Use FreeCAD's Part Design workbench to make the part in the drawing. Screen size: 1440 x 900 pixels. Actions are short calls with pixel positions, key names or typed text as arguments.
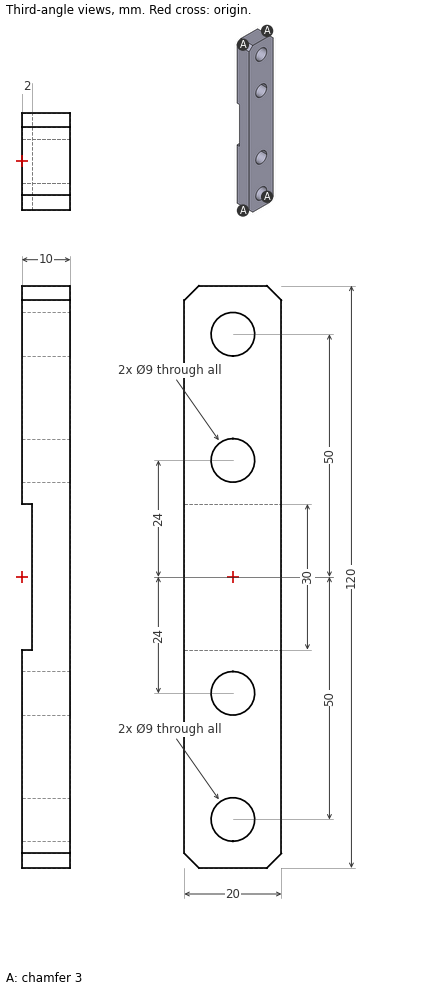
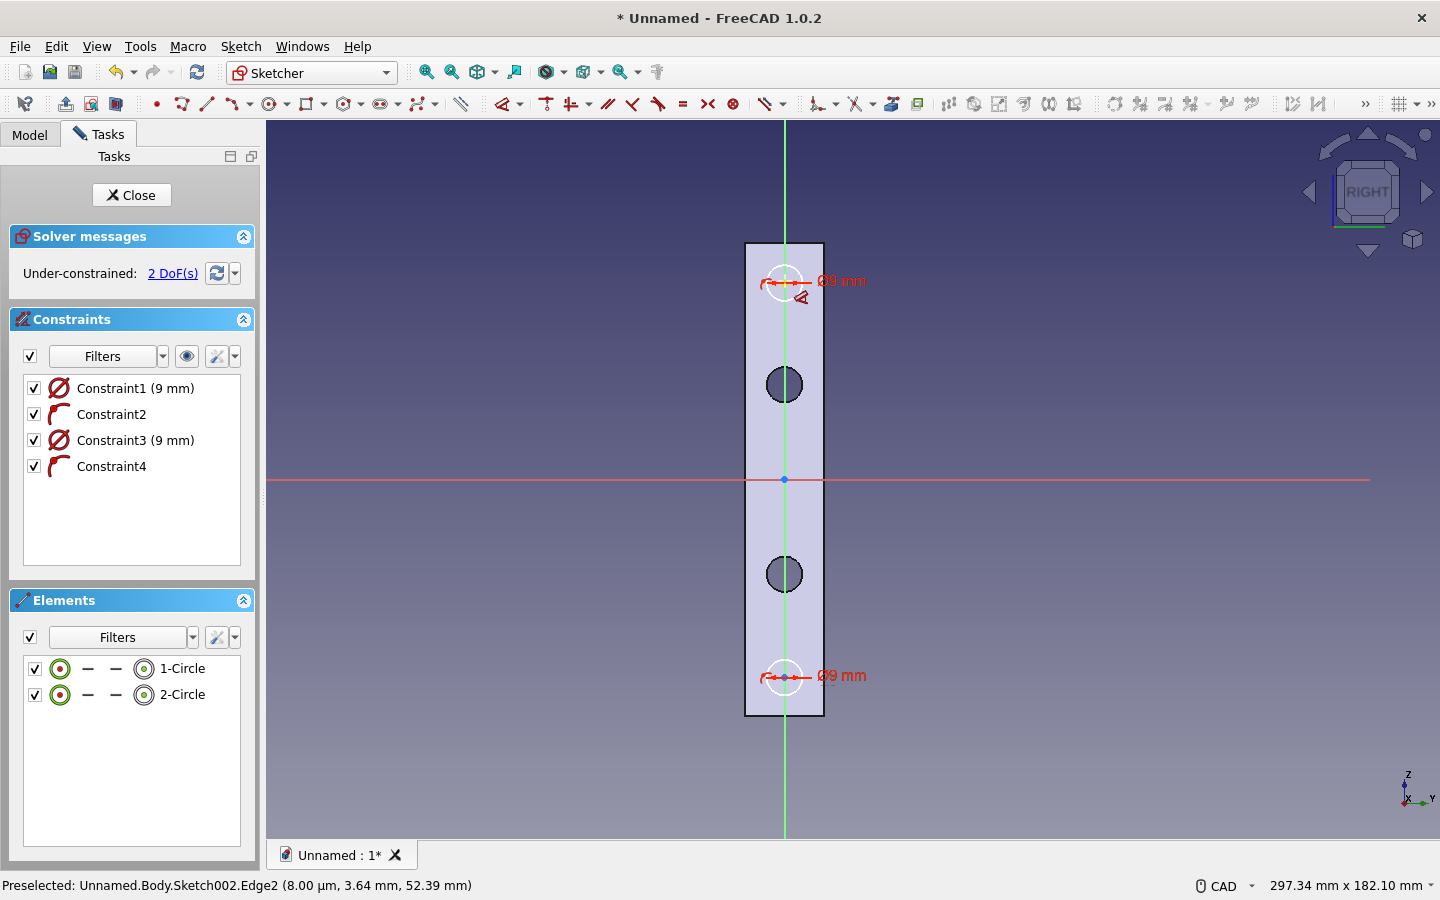
click(785, 678)
click(819, 579)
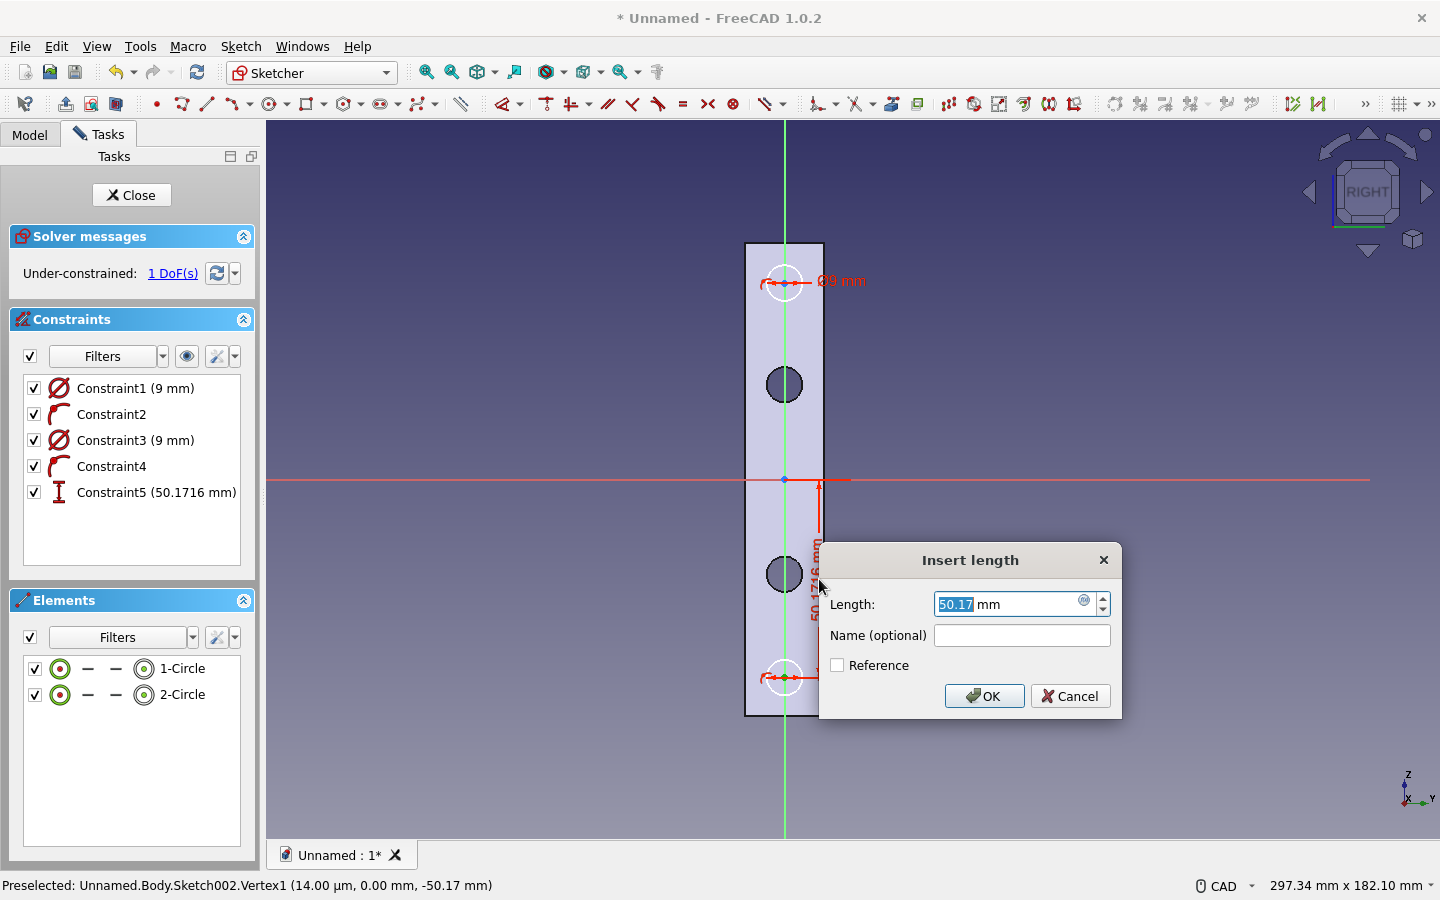
text(50)
key(Return)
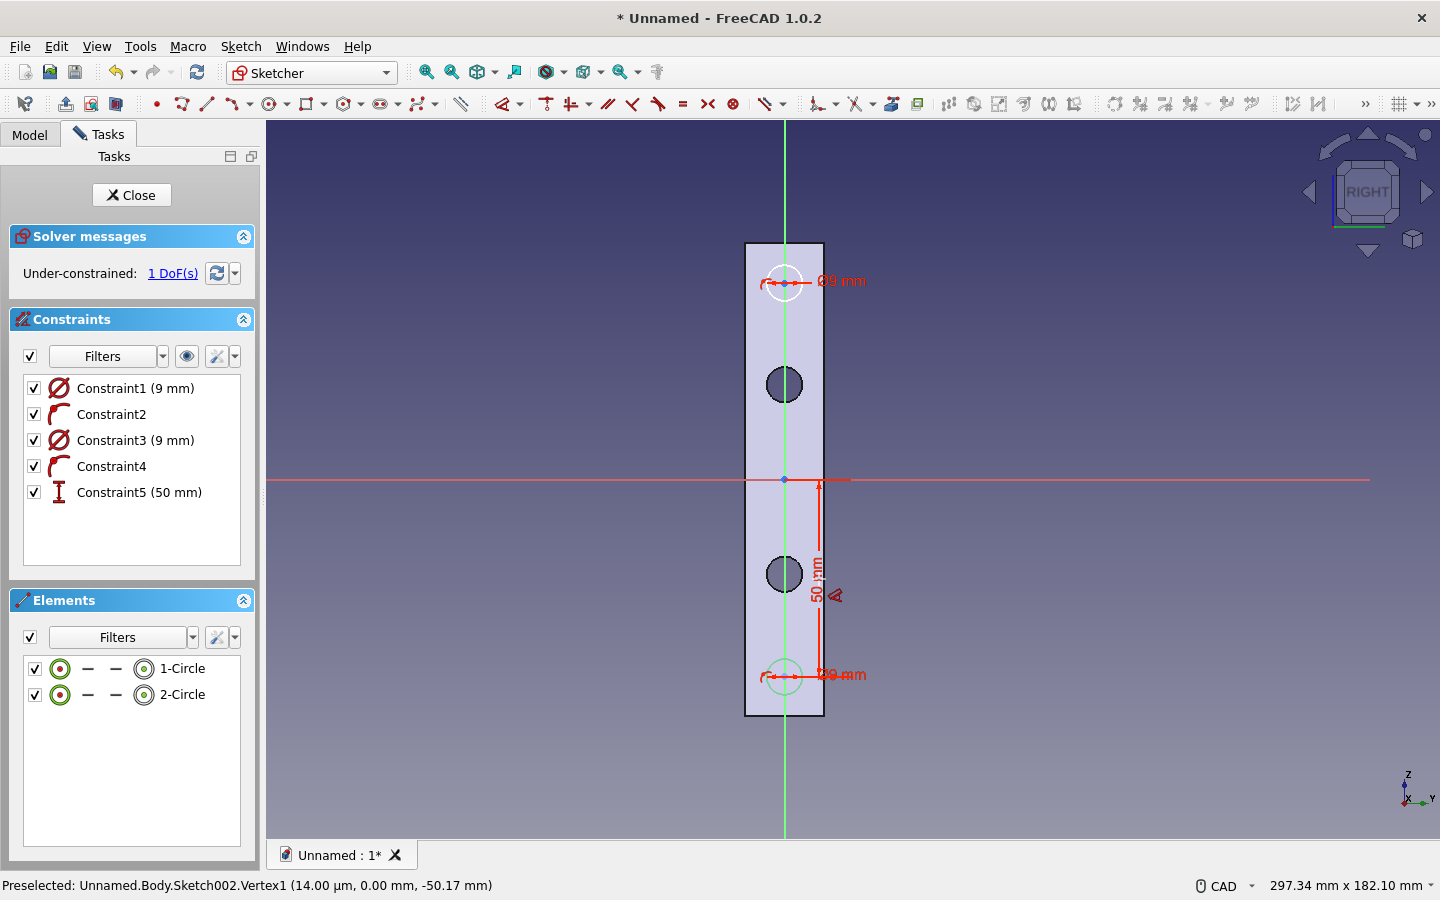
click(785, 283)
click(819, 381)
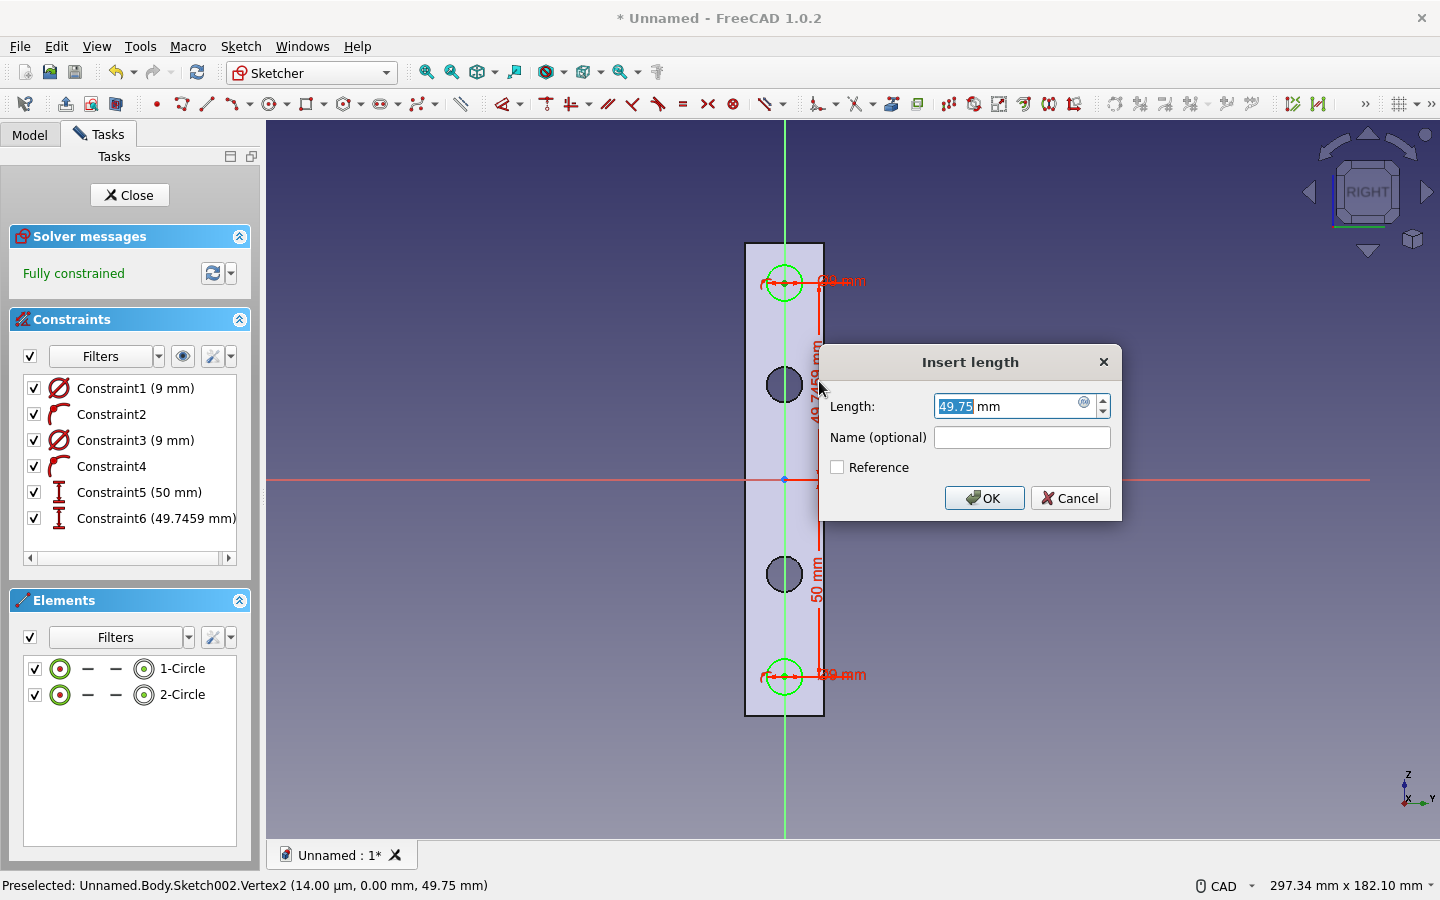
text(50)
key(Return)
key(Escape)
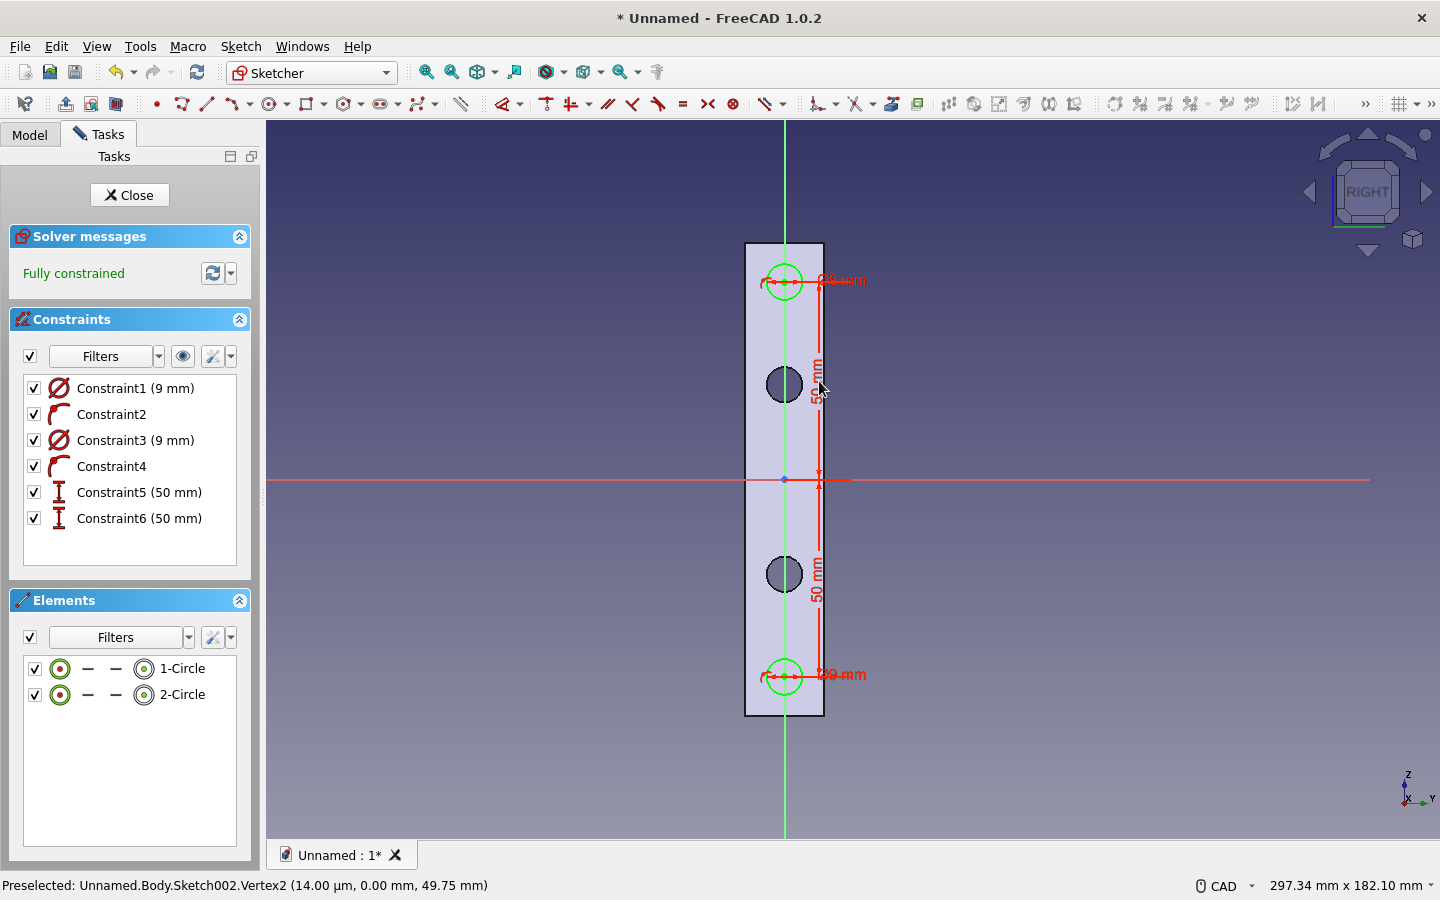
click(130, 195)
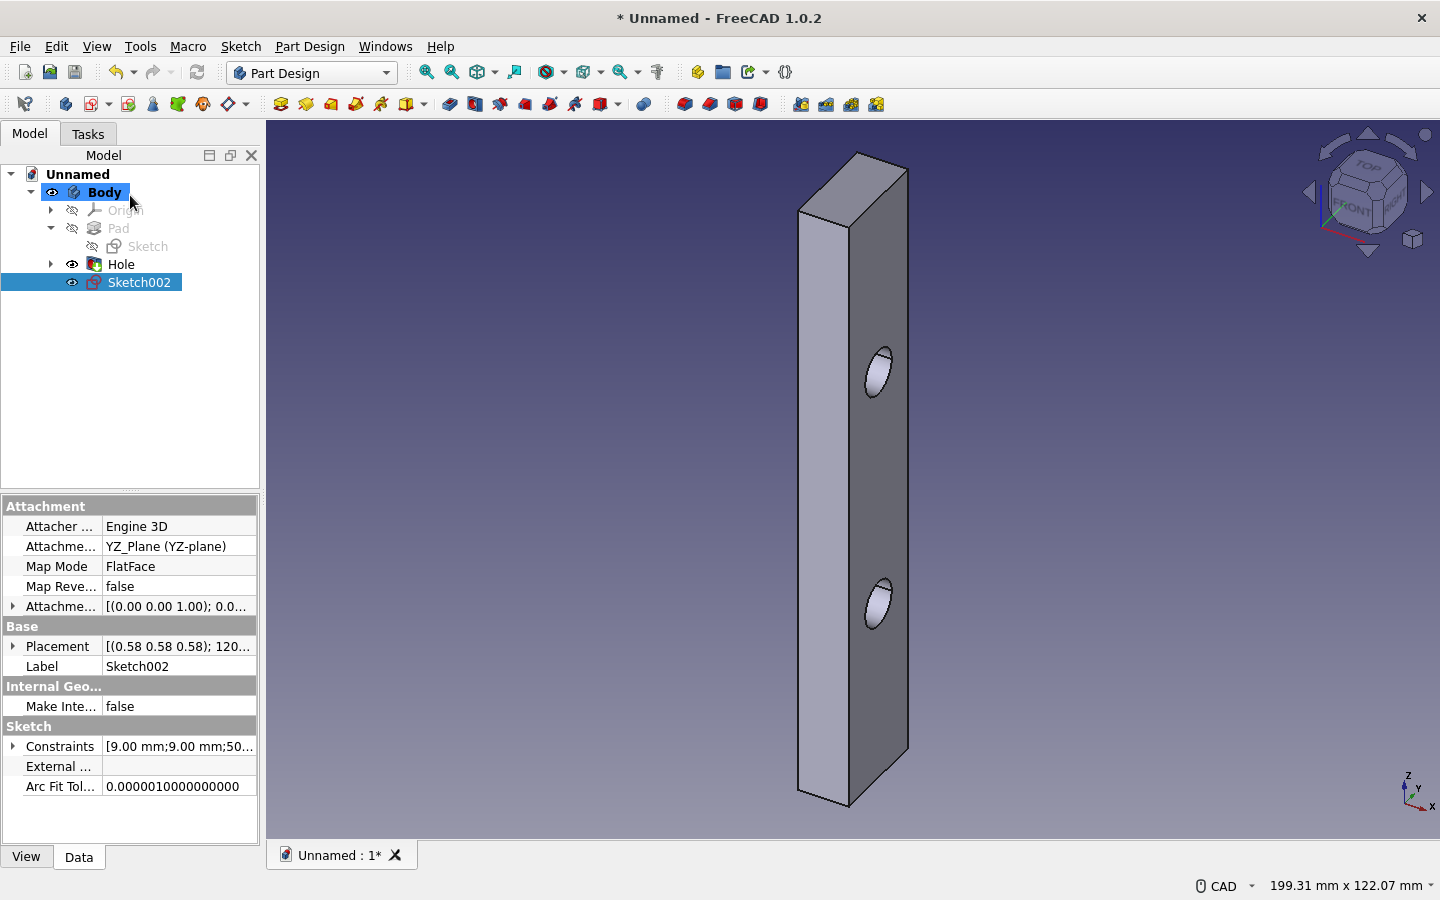
click(475, 104)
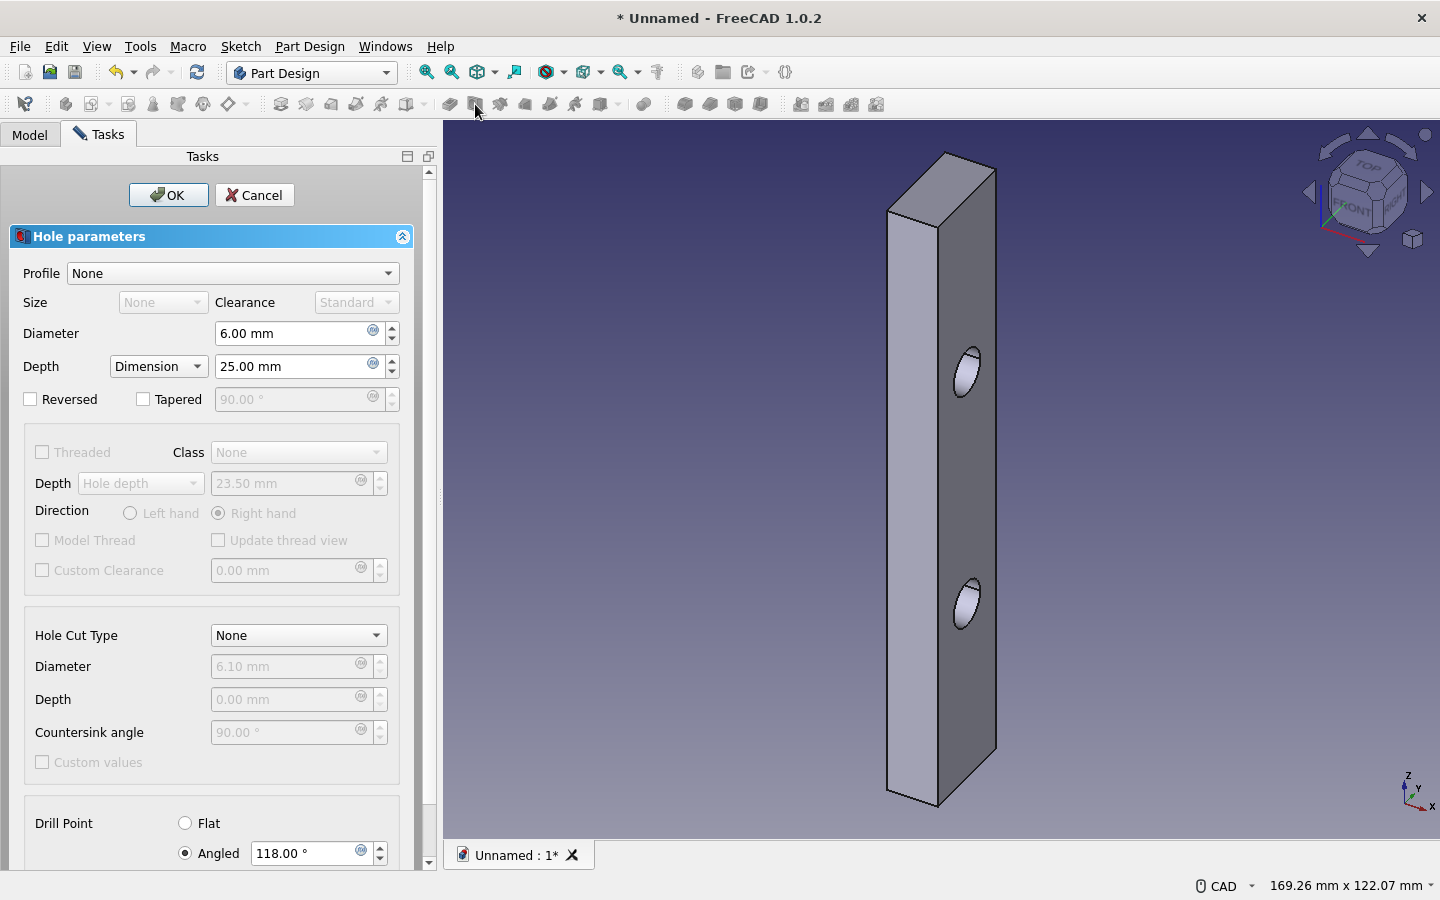
triple_click(300, 334)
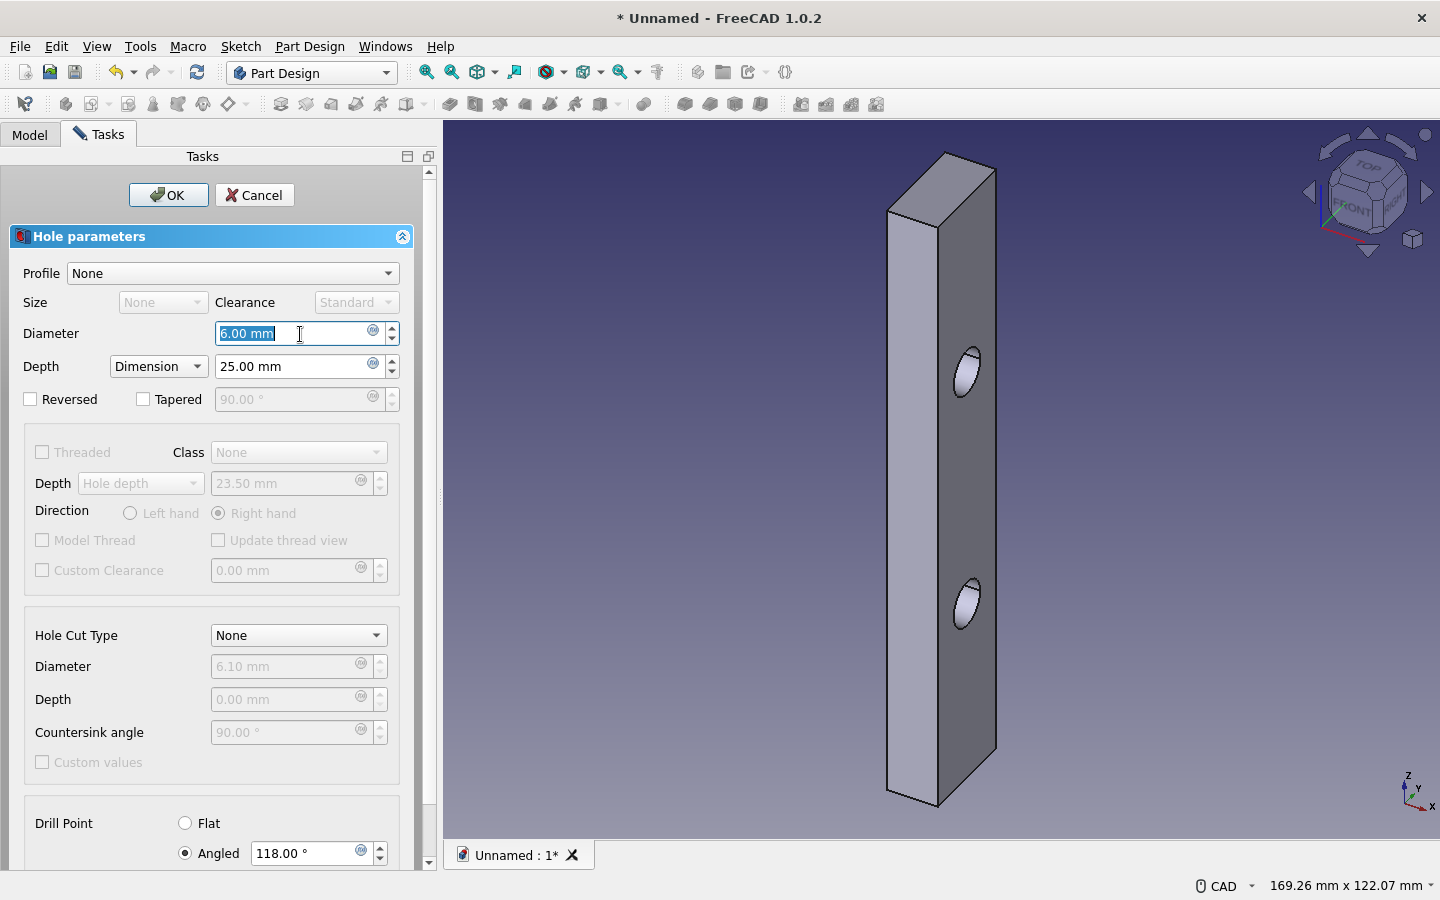
text(9)
key(Tab)